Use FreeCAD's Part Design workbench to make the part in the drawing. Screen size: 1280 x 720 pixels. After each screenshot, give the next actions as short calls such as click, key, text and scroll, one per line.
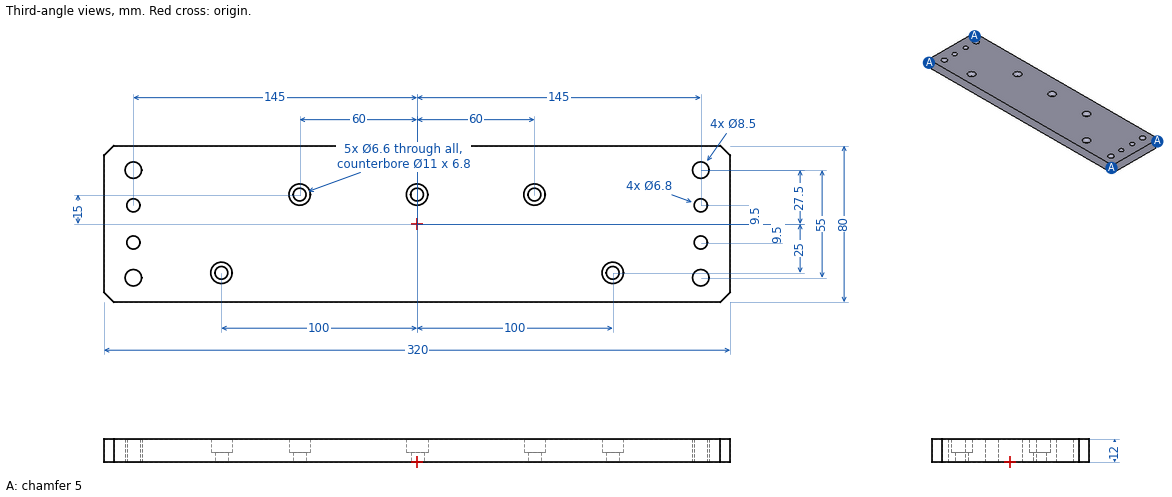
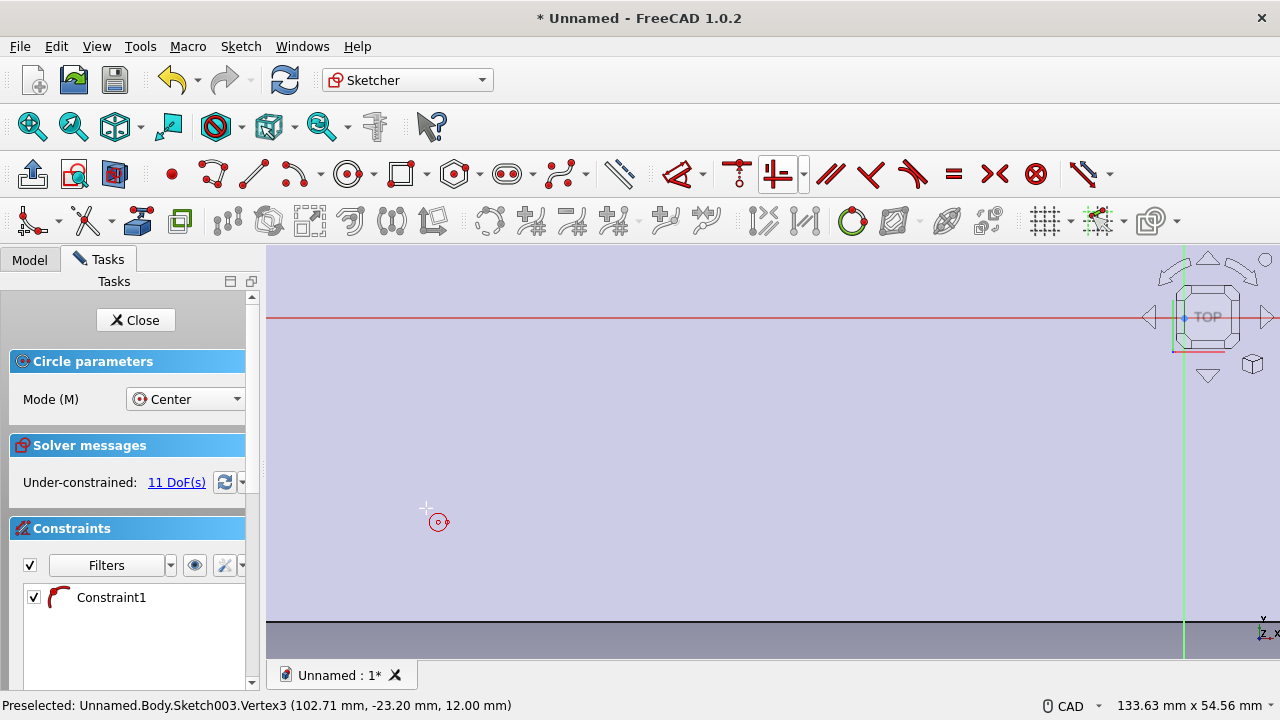
click(425, 508)
click(443, 490)
key(Escape)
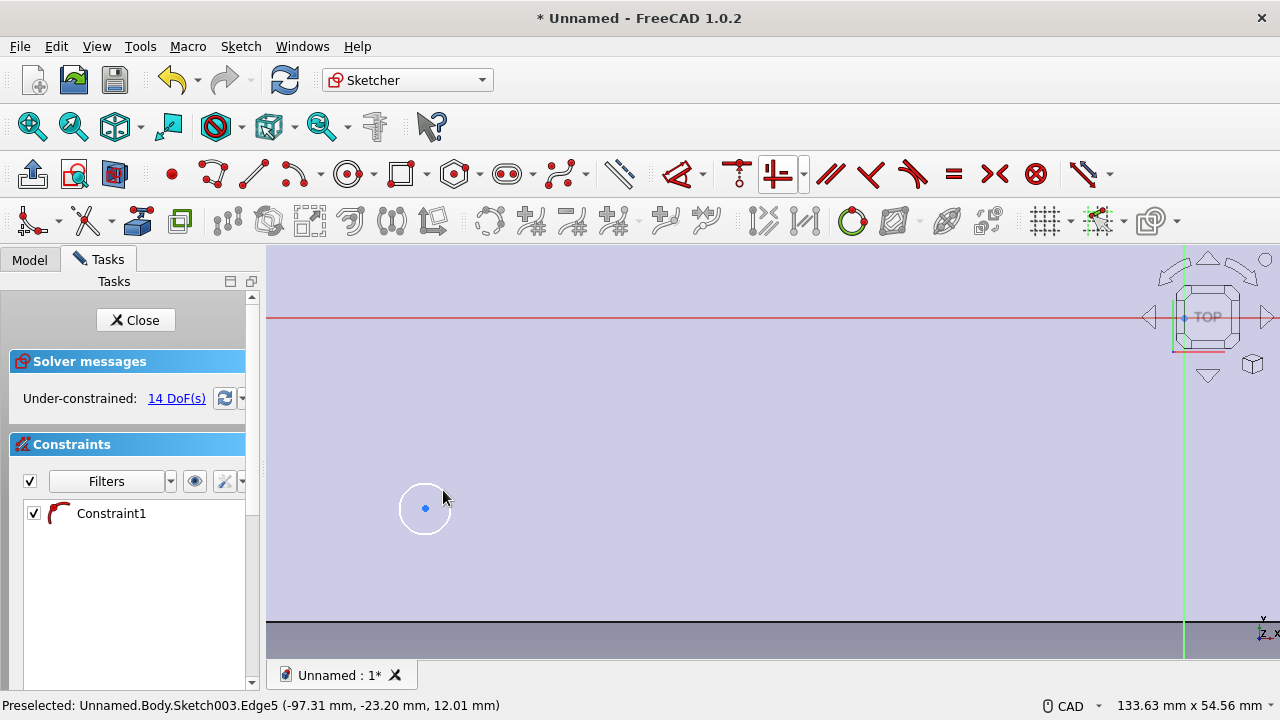
scroll(425, 508, down, 5)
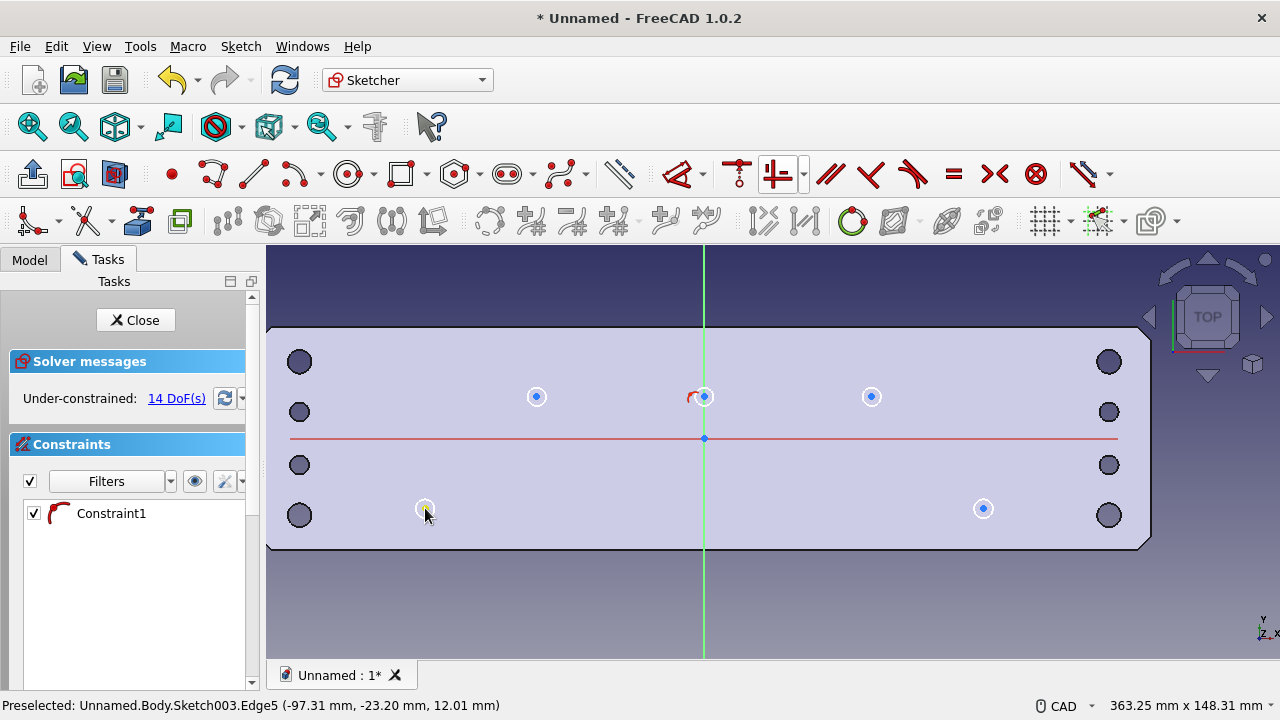
scroll(543, 390, up, 3)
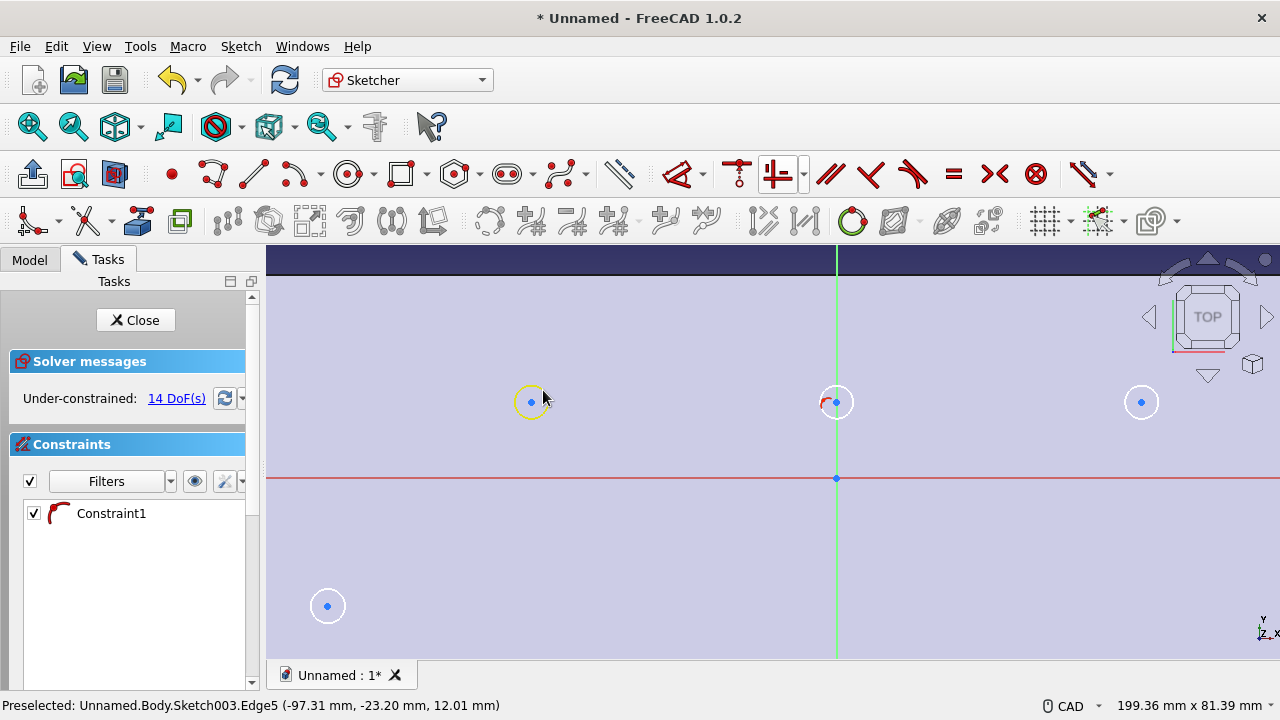
click(543, 390)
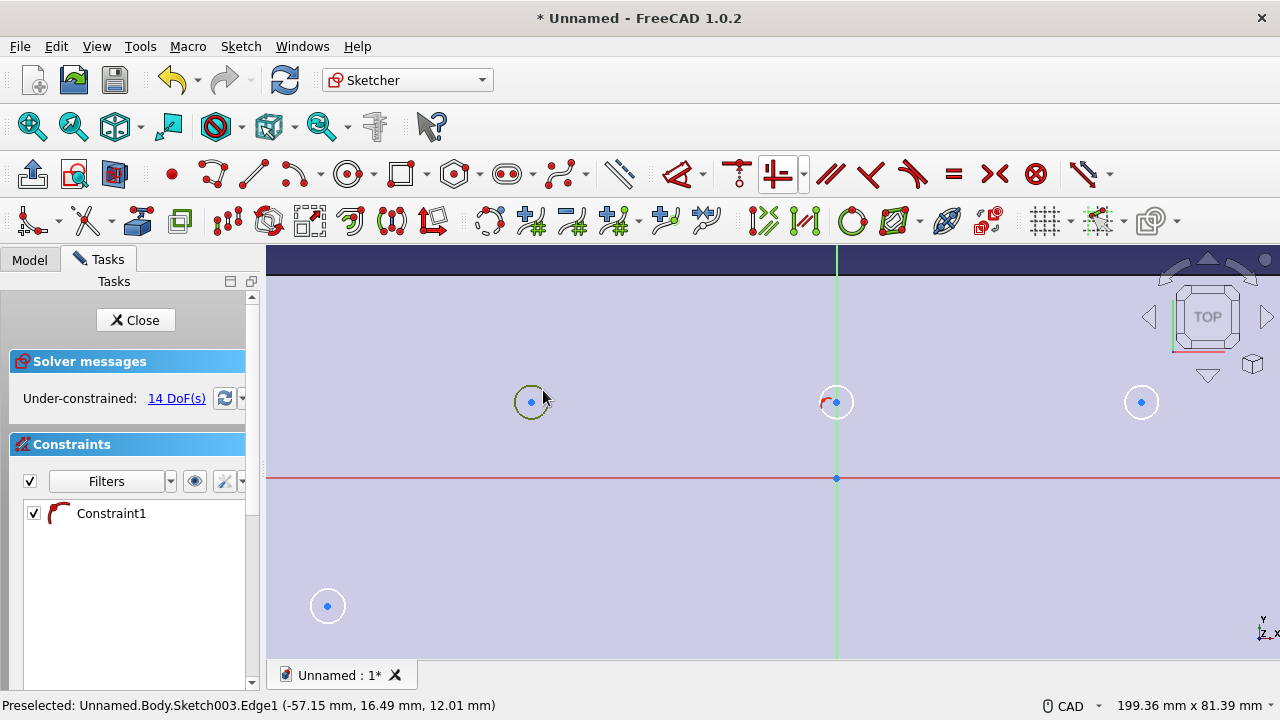
click(848, 391)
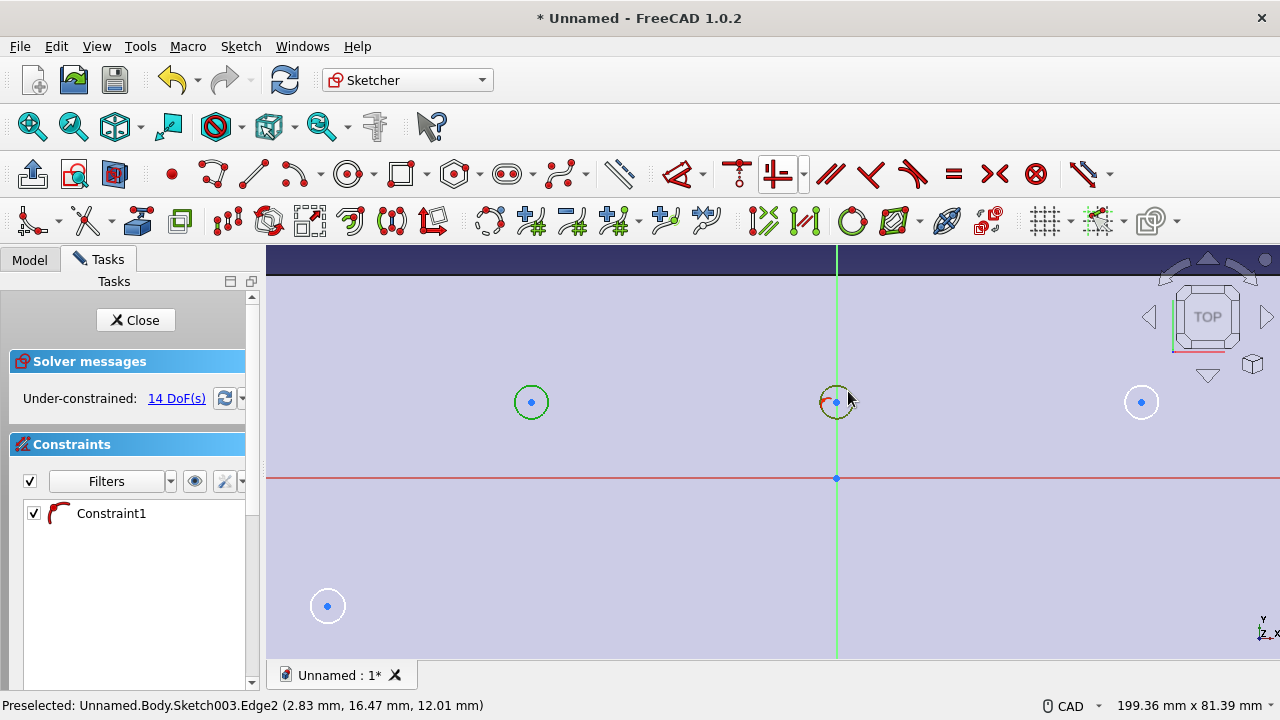
scroll(544, 389, down, 3)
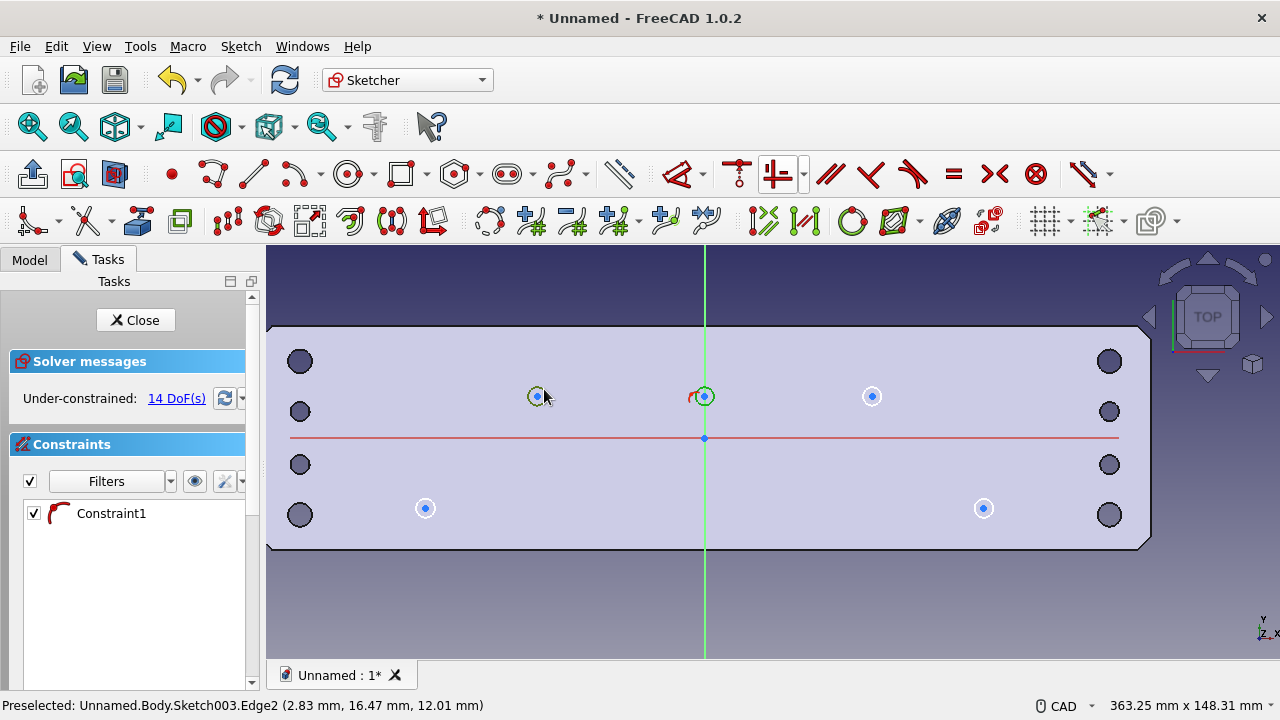
scroll(879, 390, up, 3)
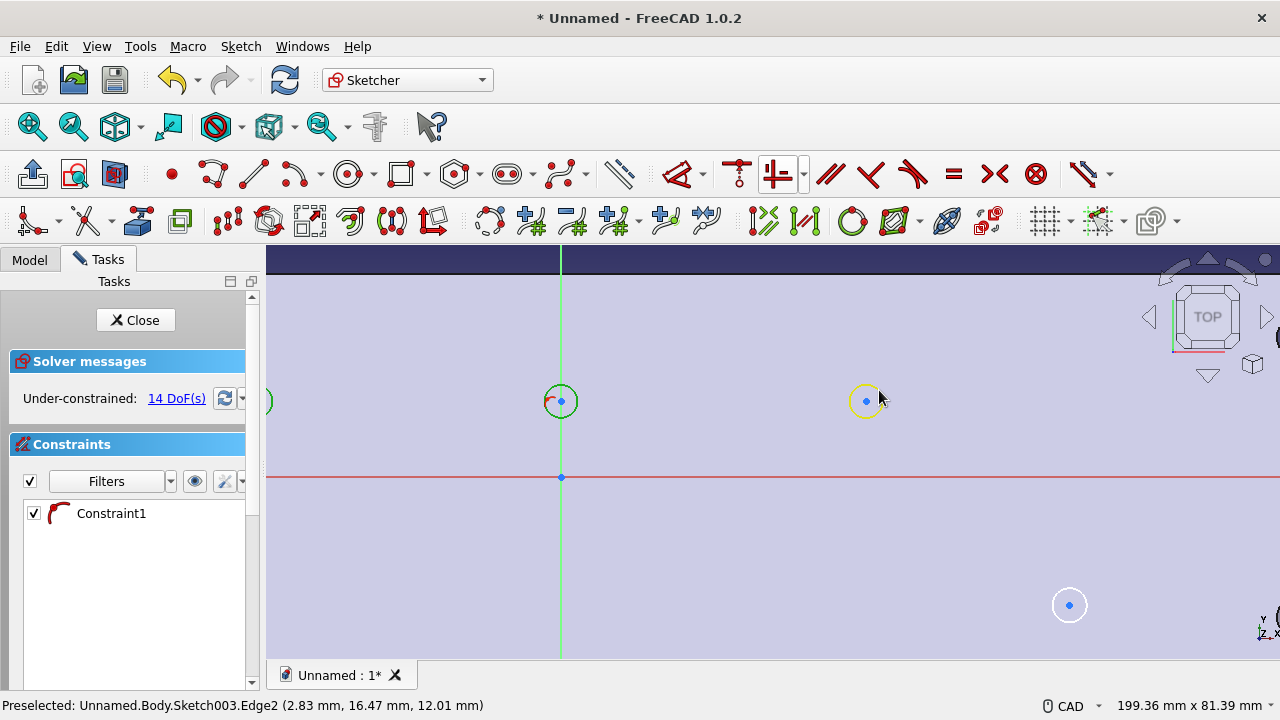
click(878, 390)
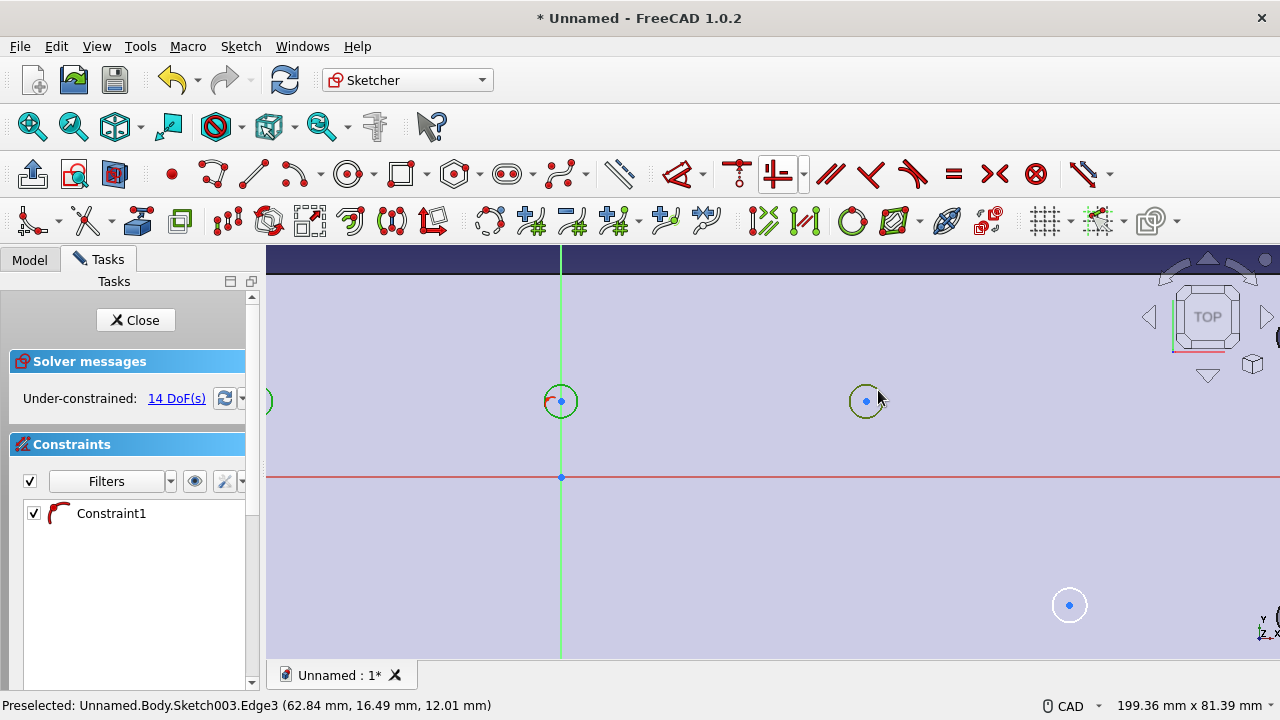
click(1082, 593)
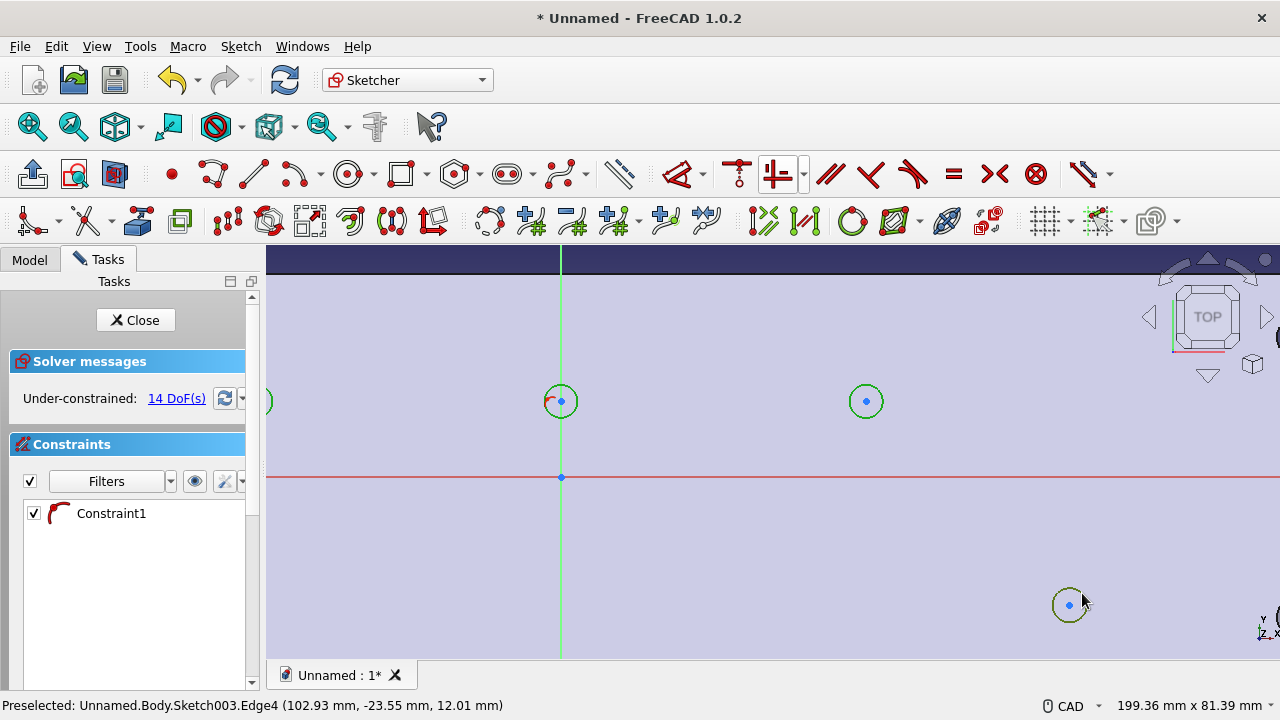
scroll(879, 390, down, 3)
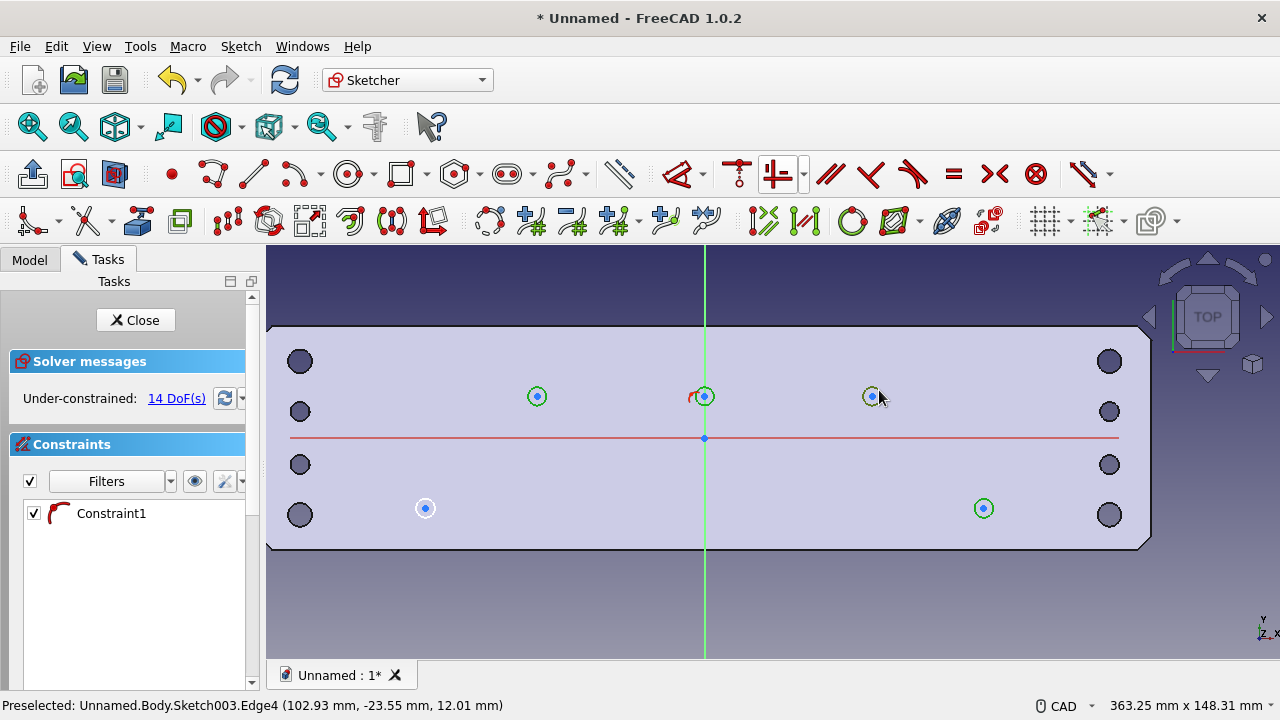
scroll(432, 502, up, 2)